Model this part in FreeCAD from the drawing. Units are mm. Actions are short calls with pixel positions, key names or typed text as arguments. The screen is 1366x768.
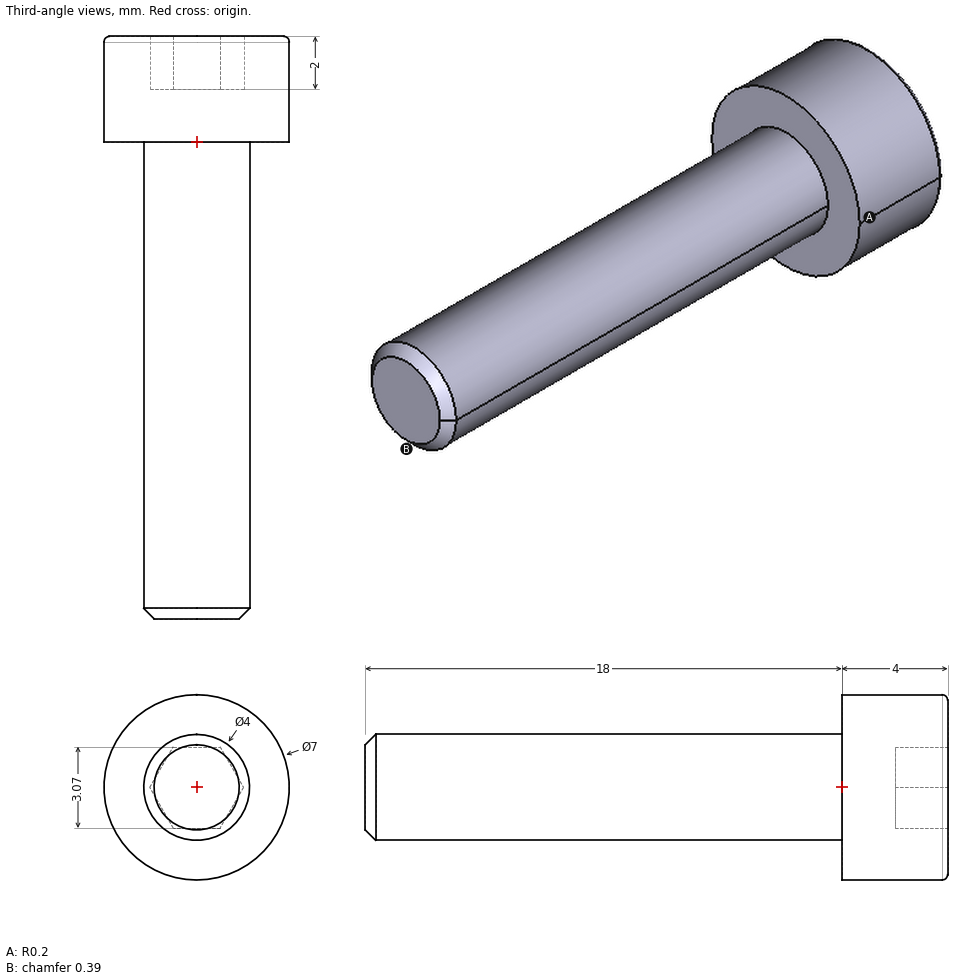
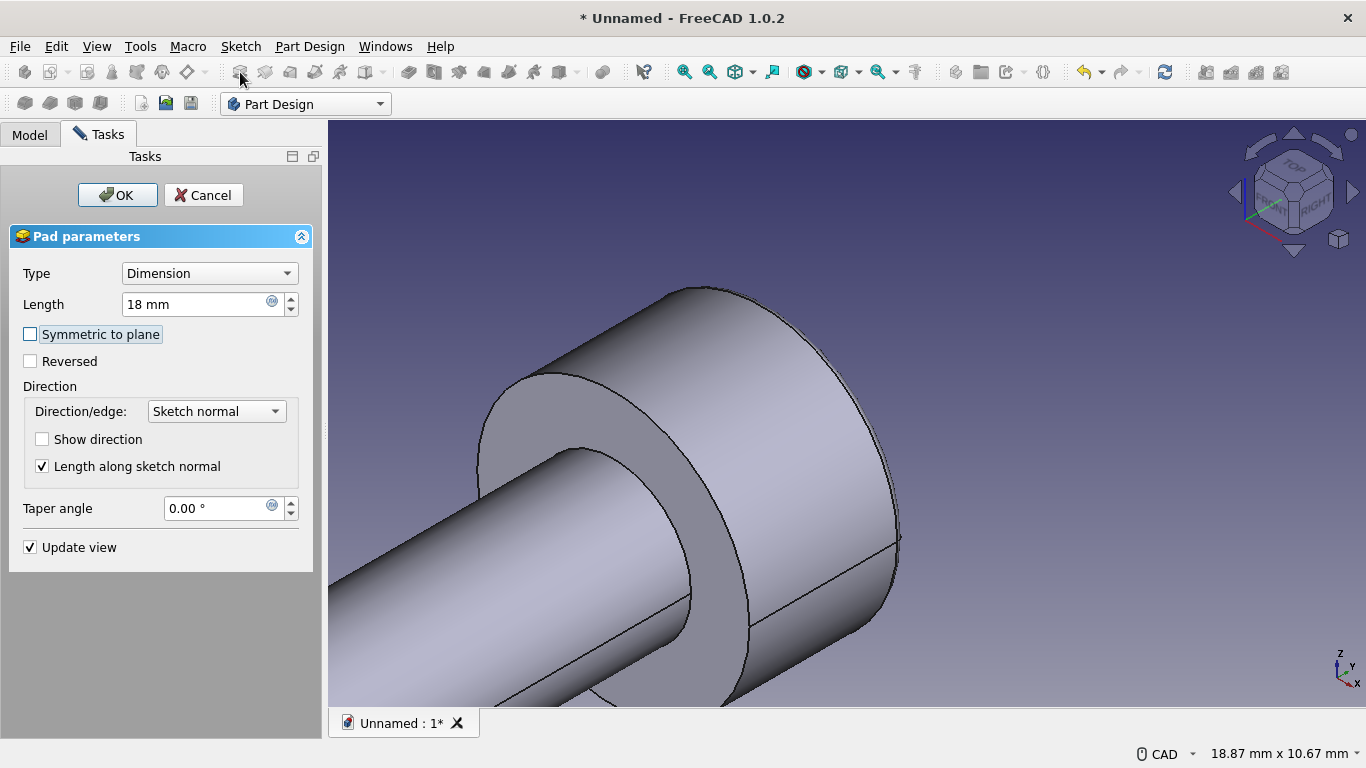
click(118, 195)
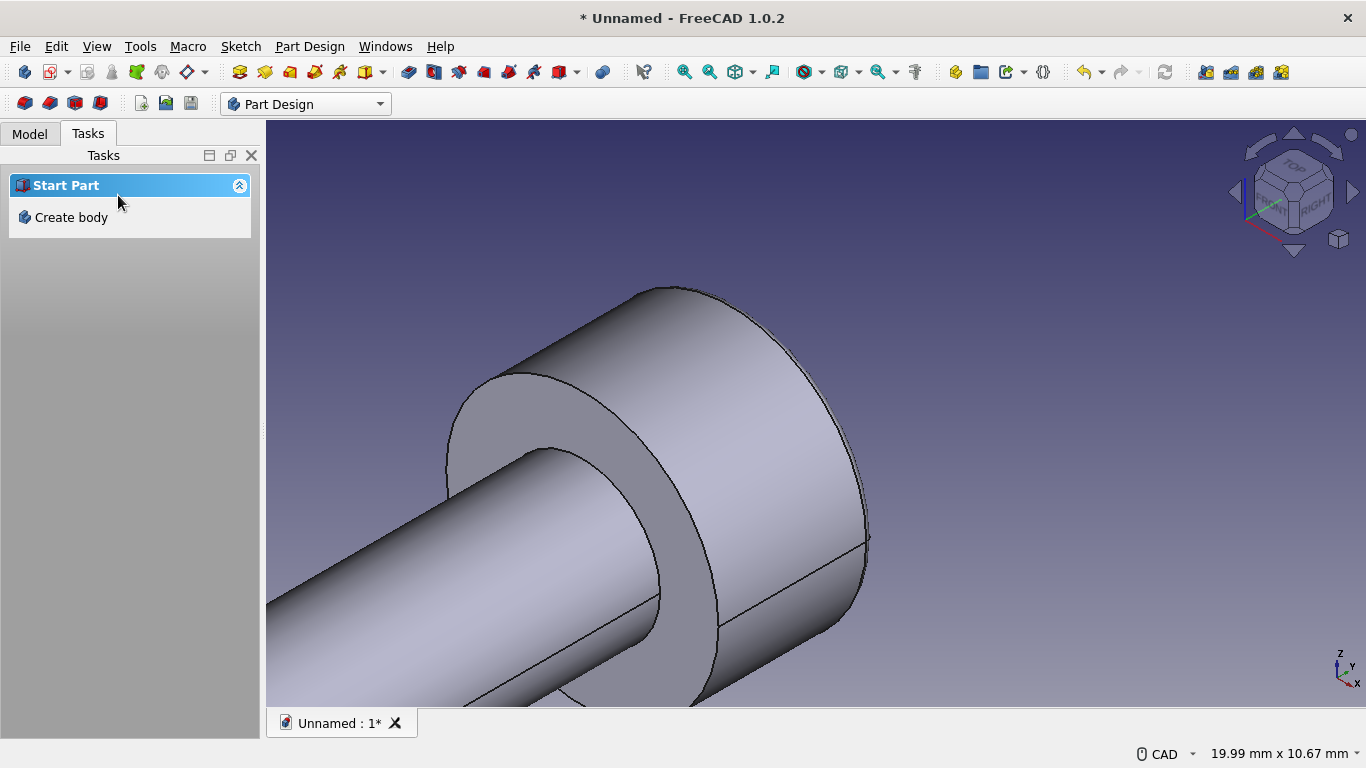
click(685, 72)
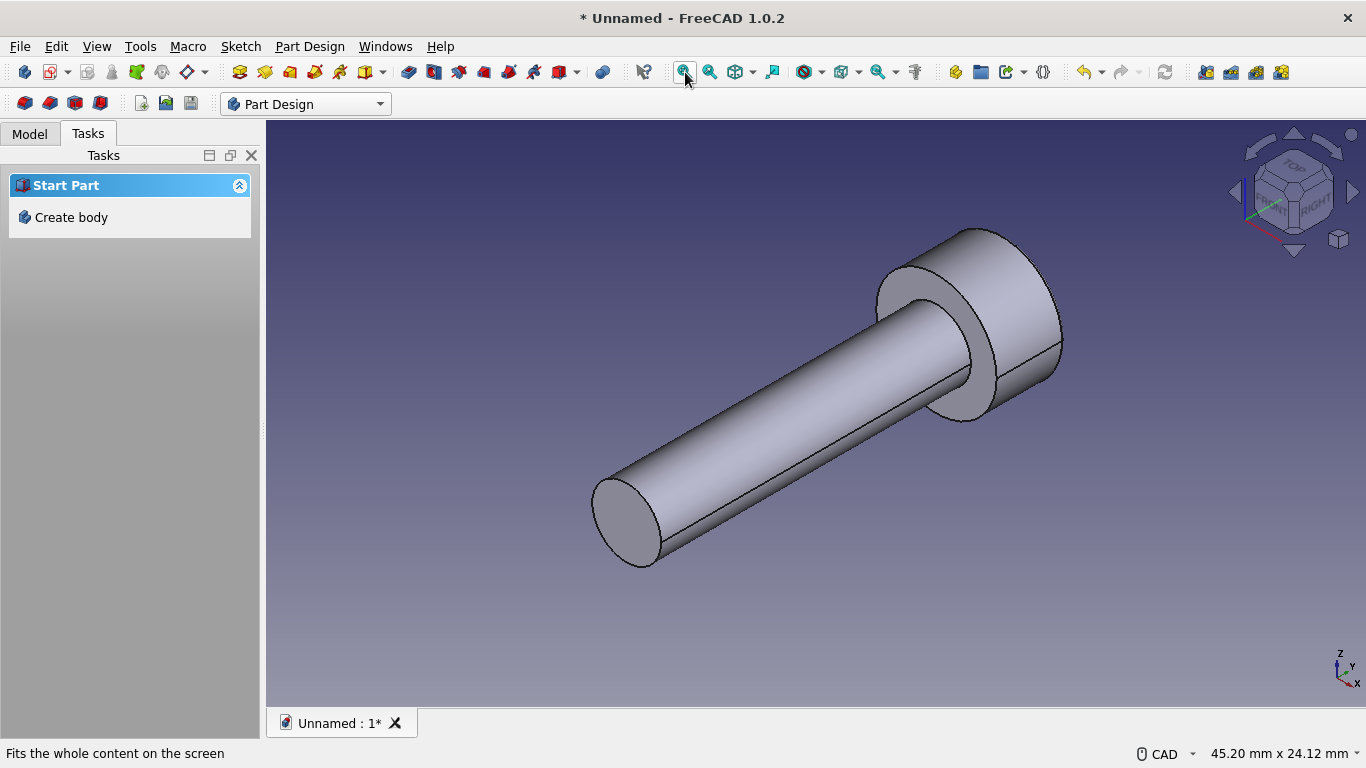
click(616, 478)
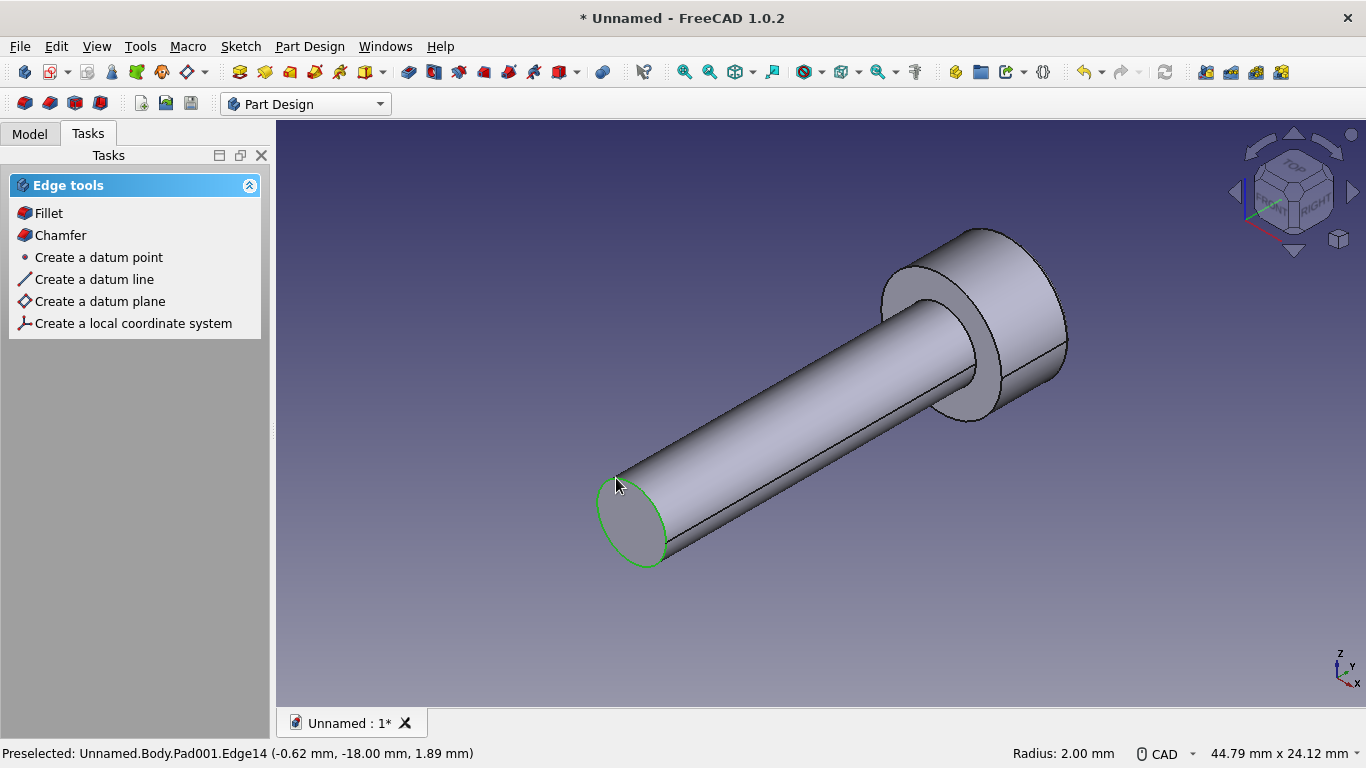
click(50, 104)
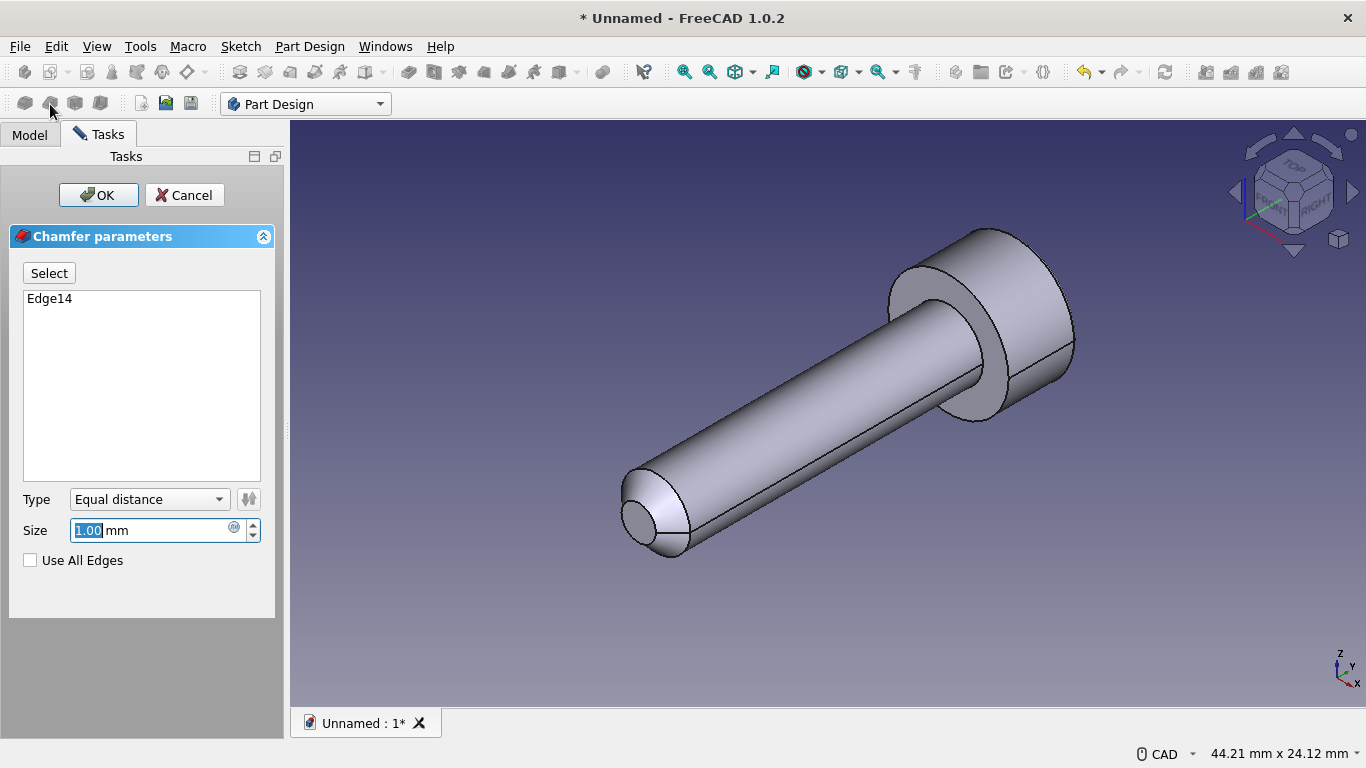
text(0.39)
key(Tab)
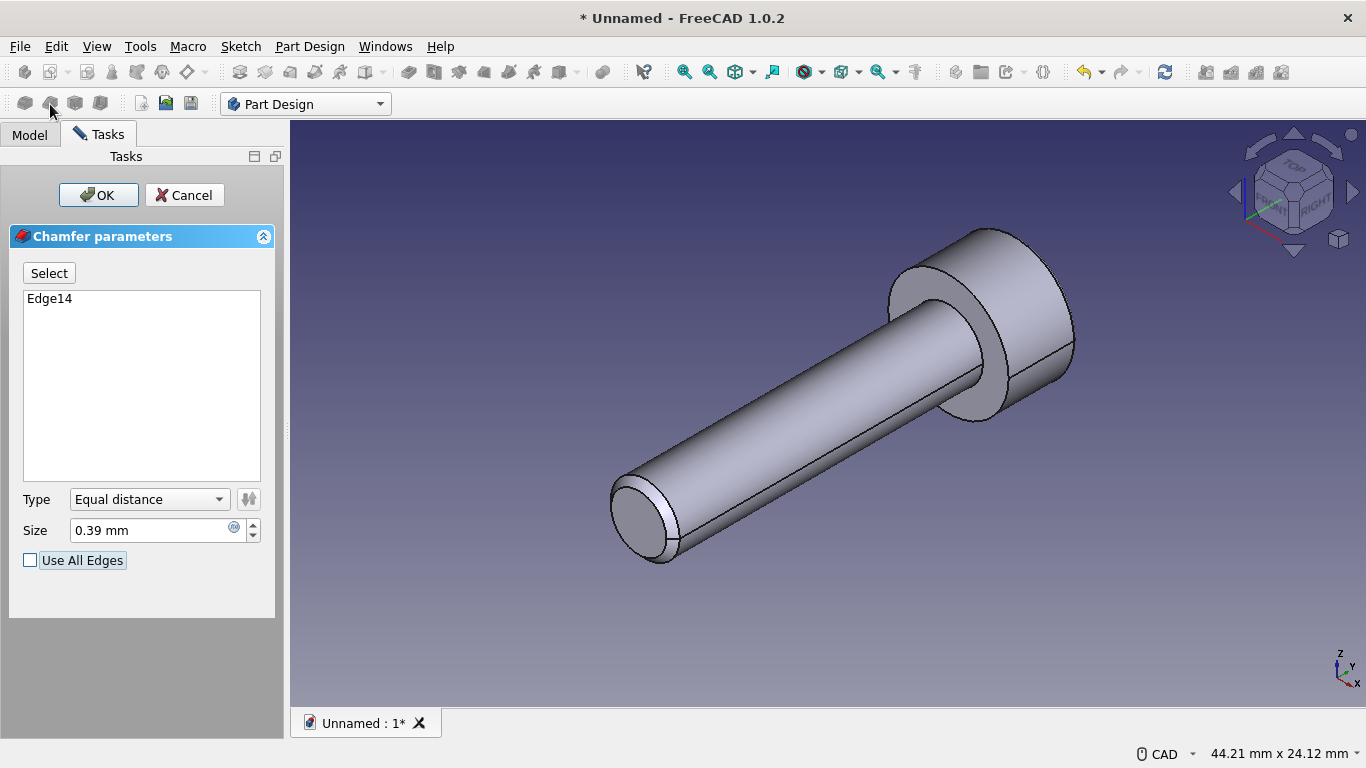
click(99, 195)